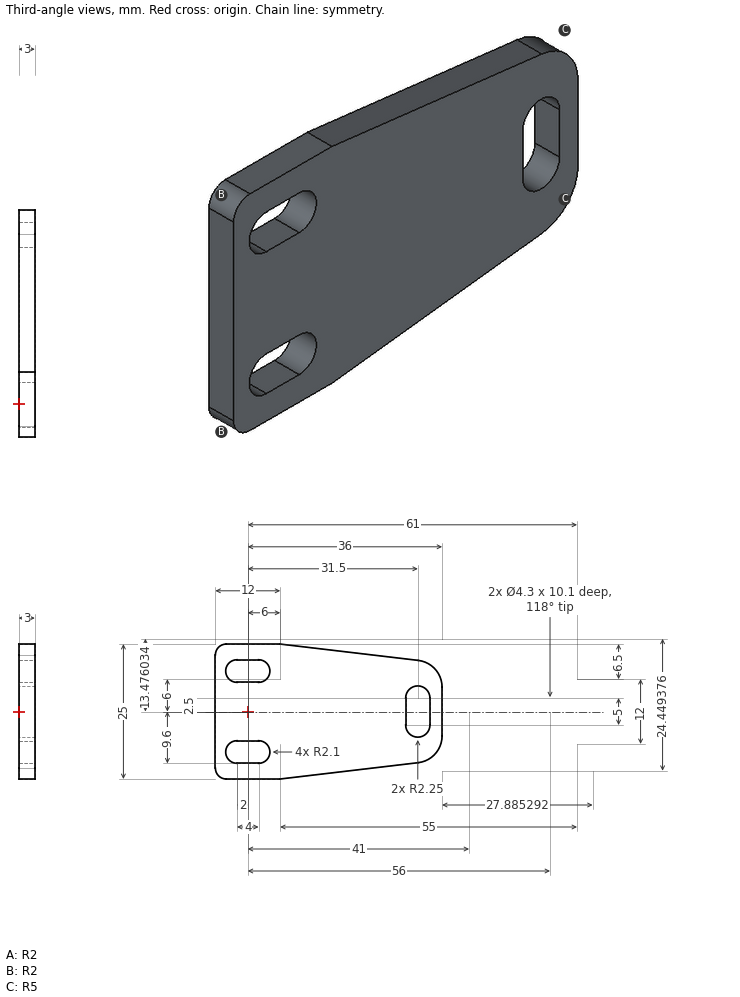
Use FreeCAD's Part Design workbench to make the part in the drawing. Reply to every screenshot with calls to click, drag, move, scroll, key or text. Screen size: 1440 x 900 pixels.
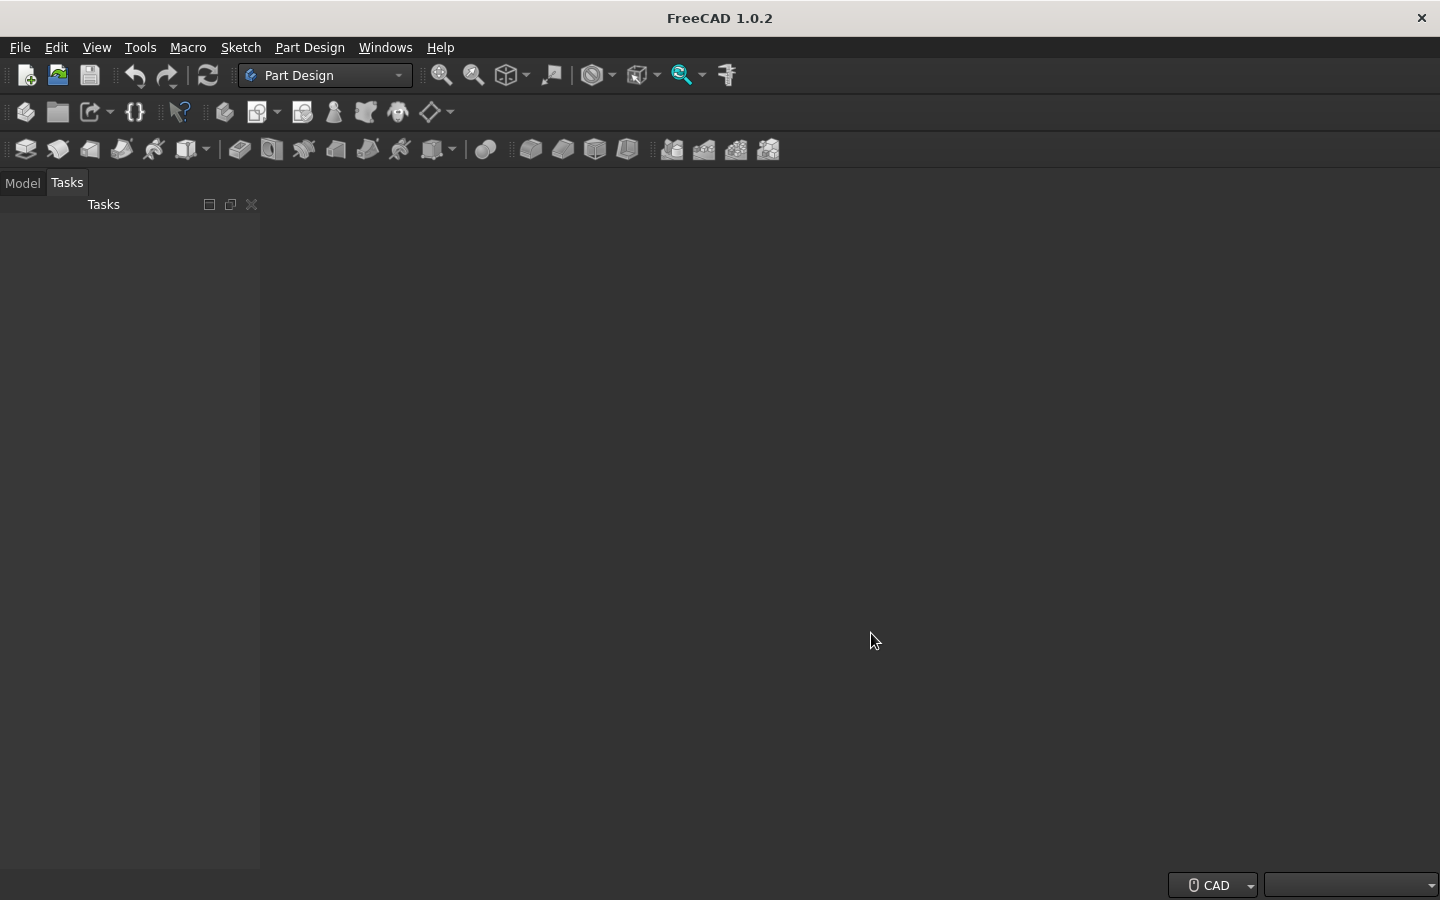
key(ctrl+n)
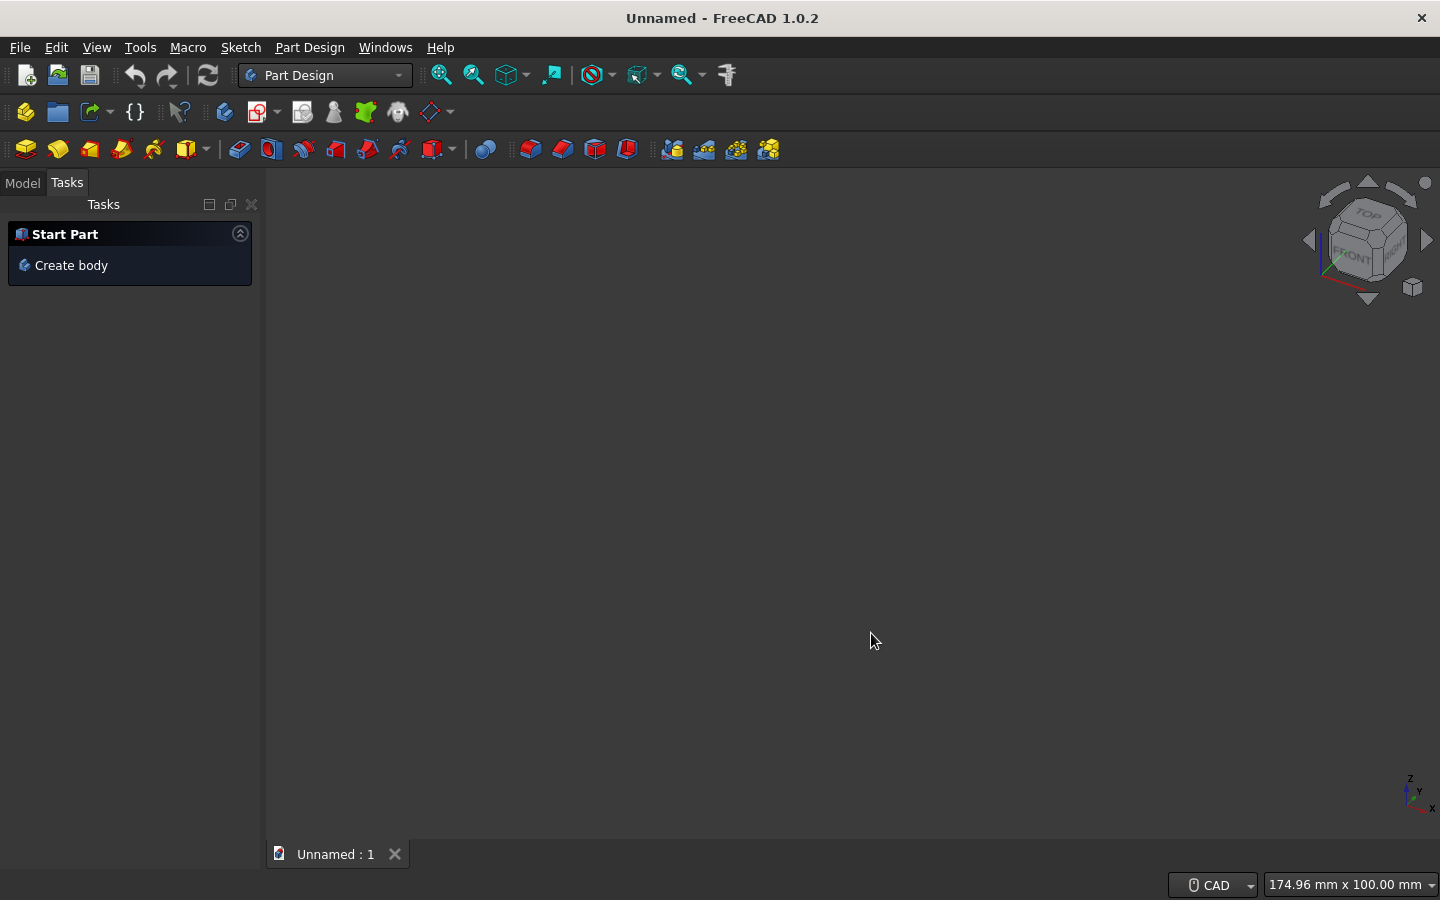
click(258, 112)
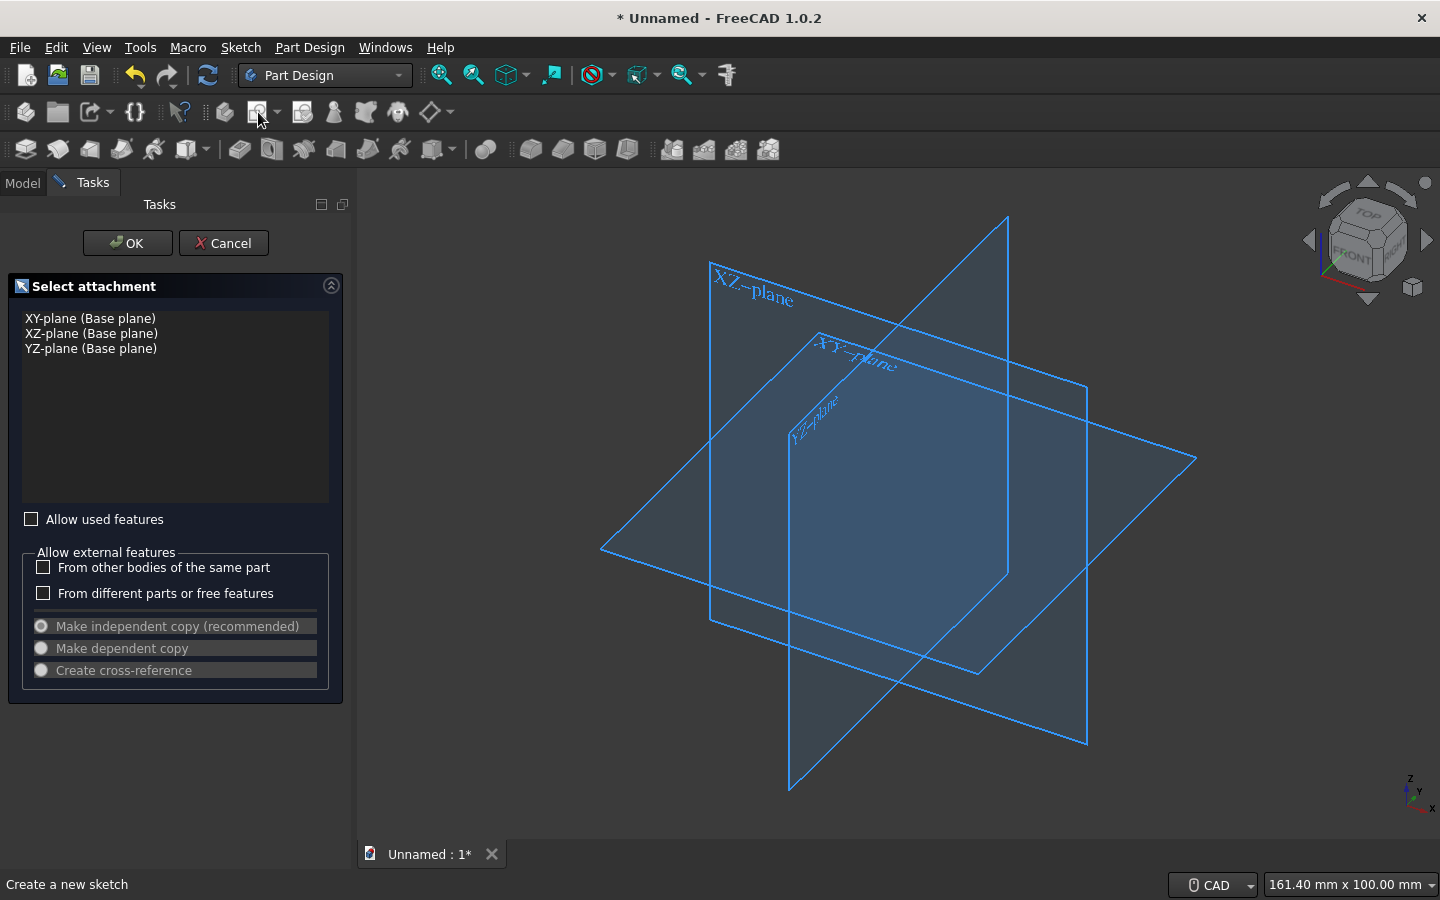
click(82, 348)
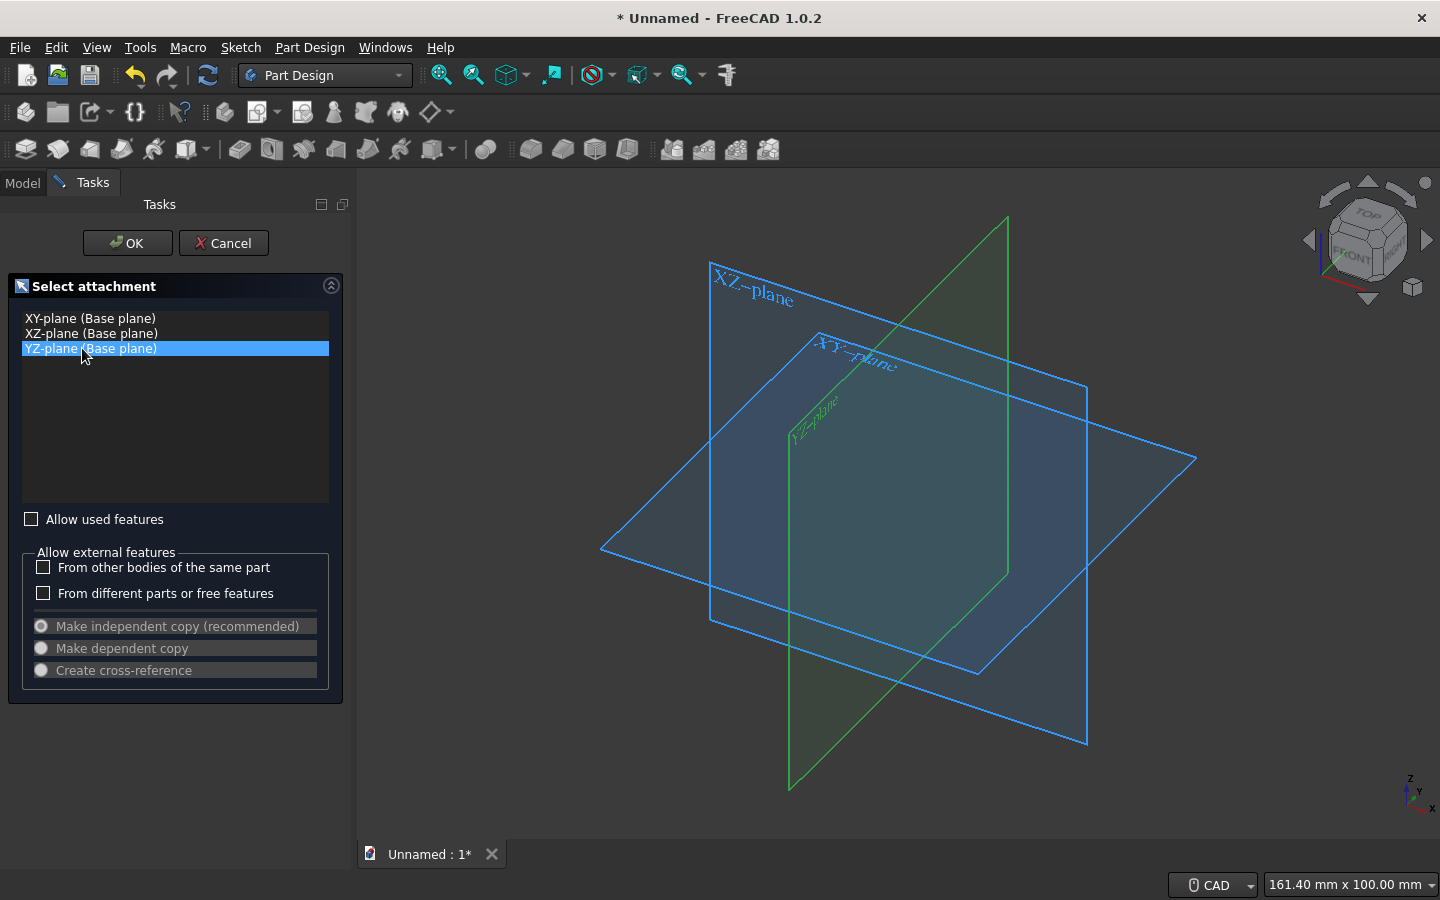
click(128, 243)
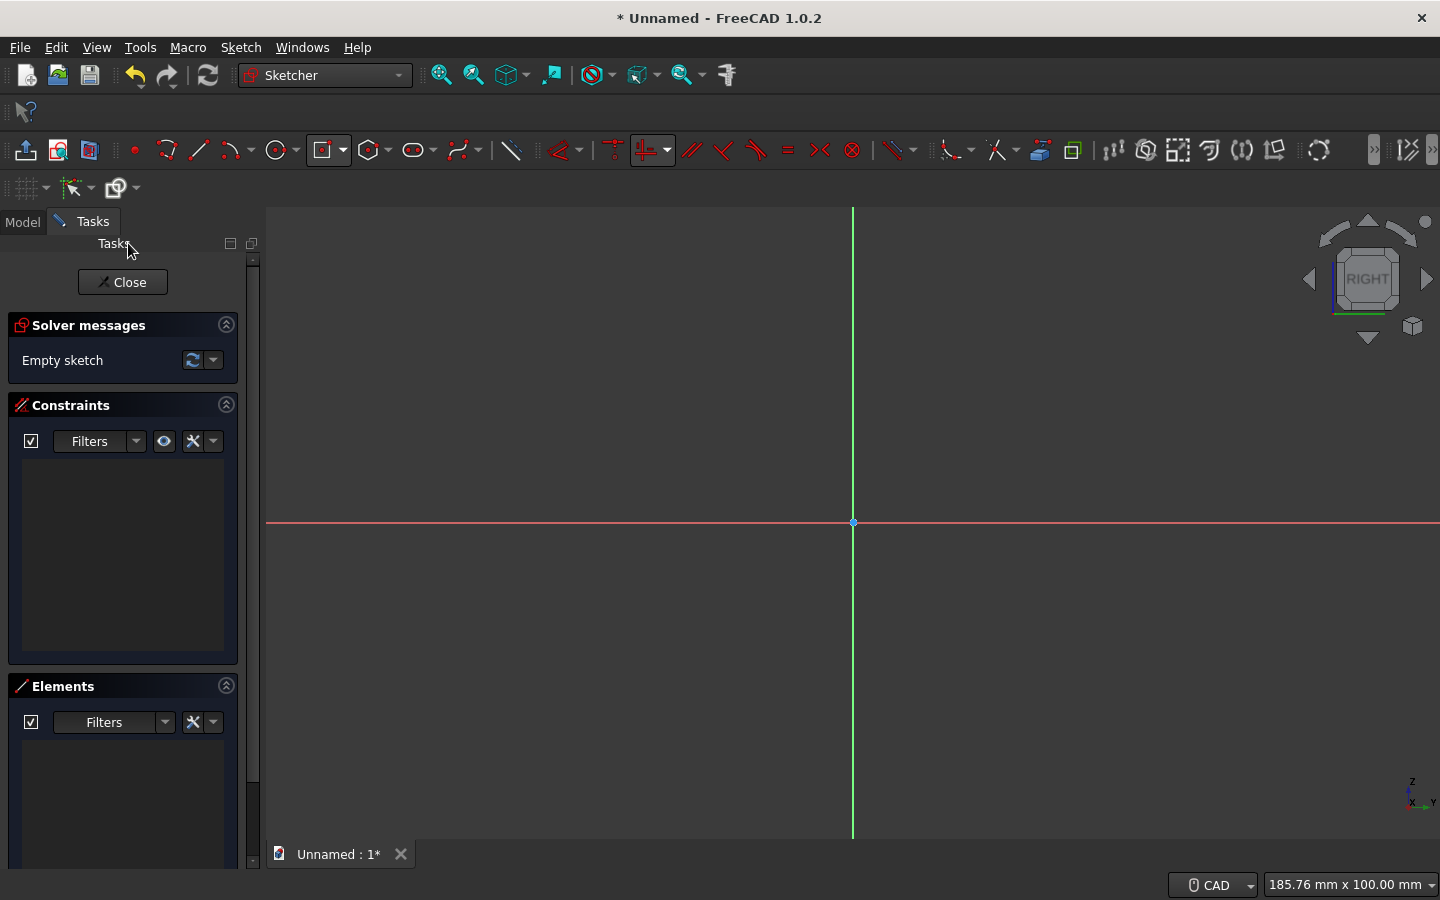
scroll(1275, 523, up, 2)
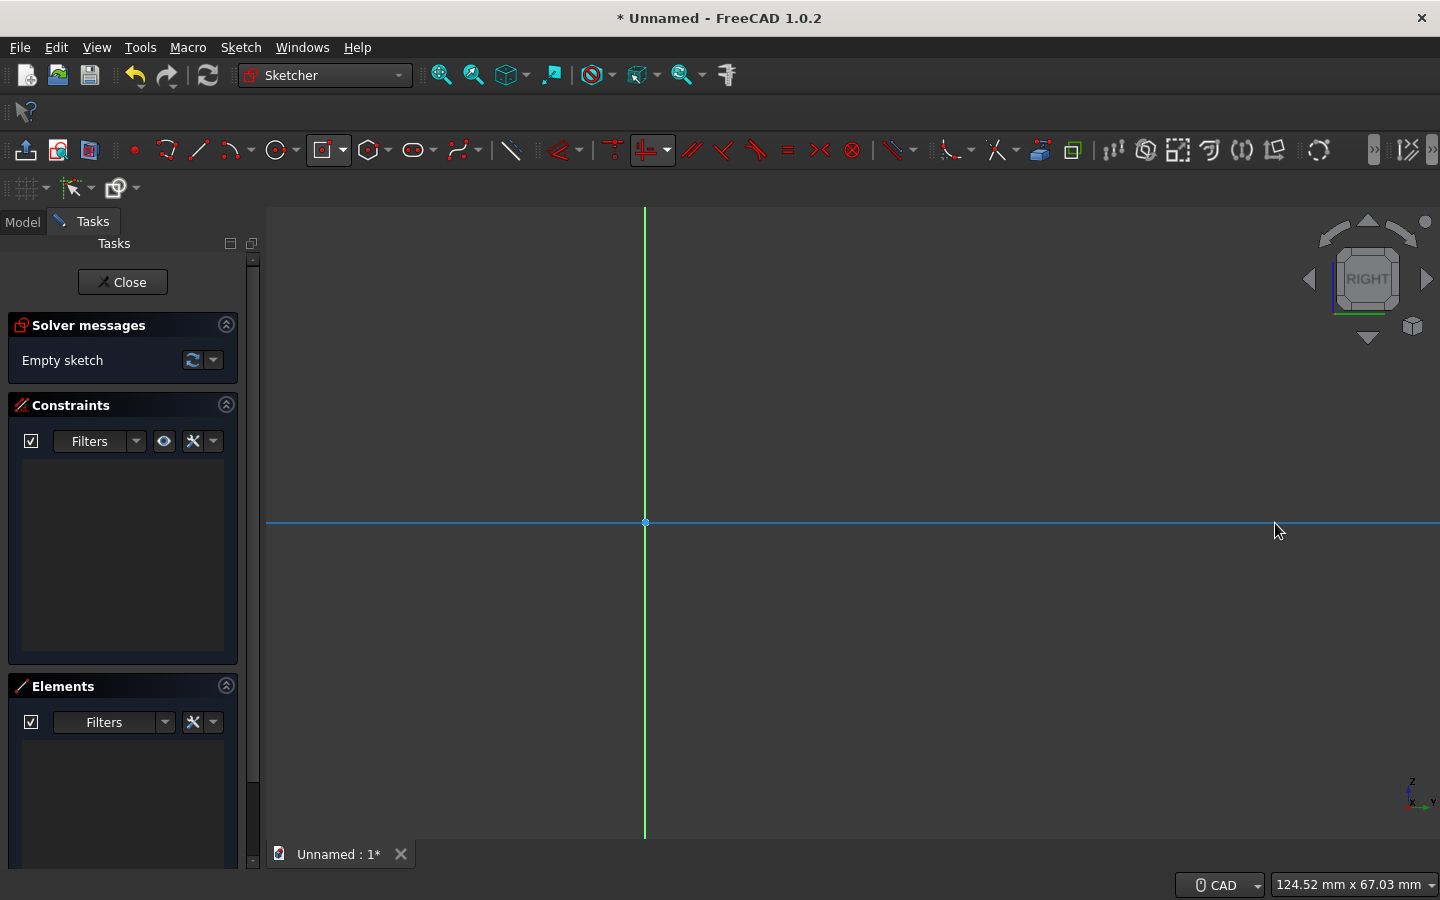
key(g)
key(m)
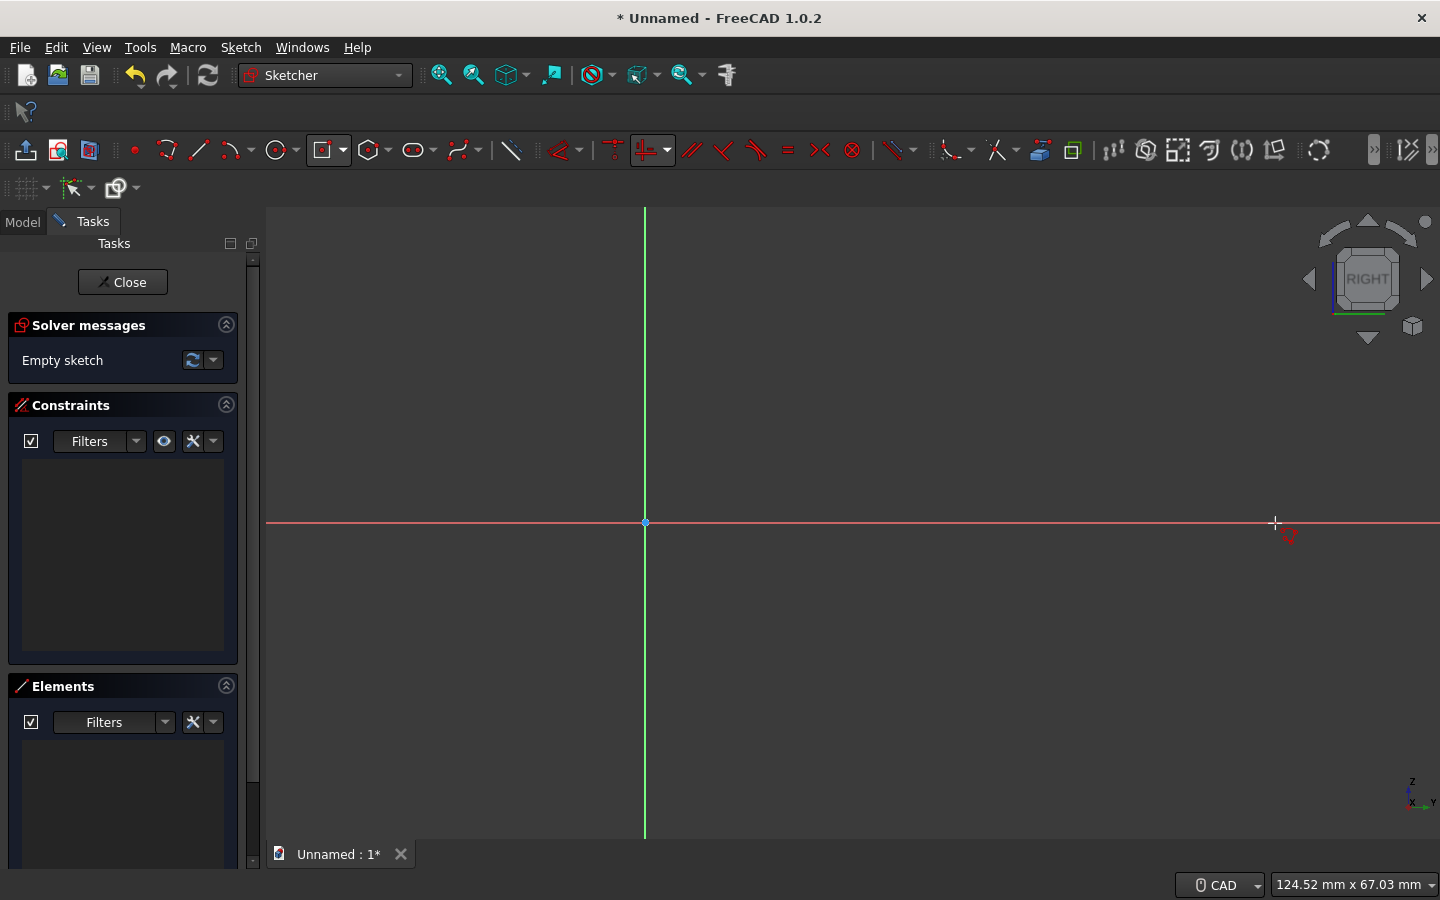
click(702, 466)
click(702, 405)
click(588, 405)
click(588, 641)
click(702, 641)
click(702, 579)
click(1220, 579)
click(1220, 466)
click(702, 467)
key(Escape)
key(Escape)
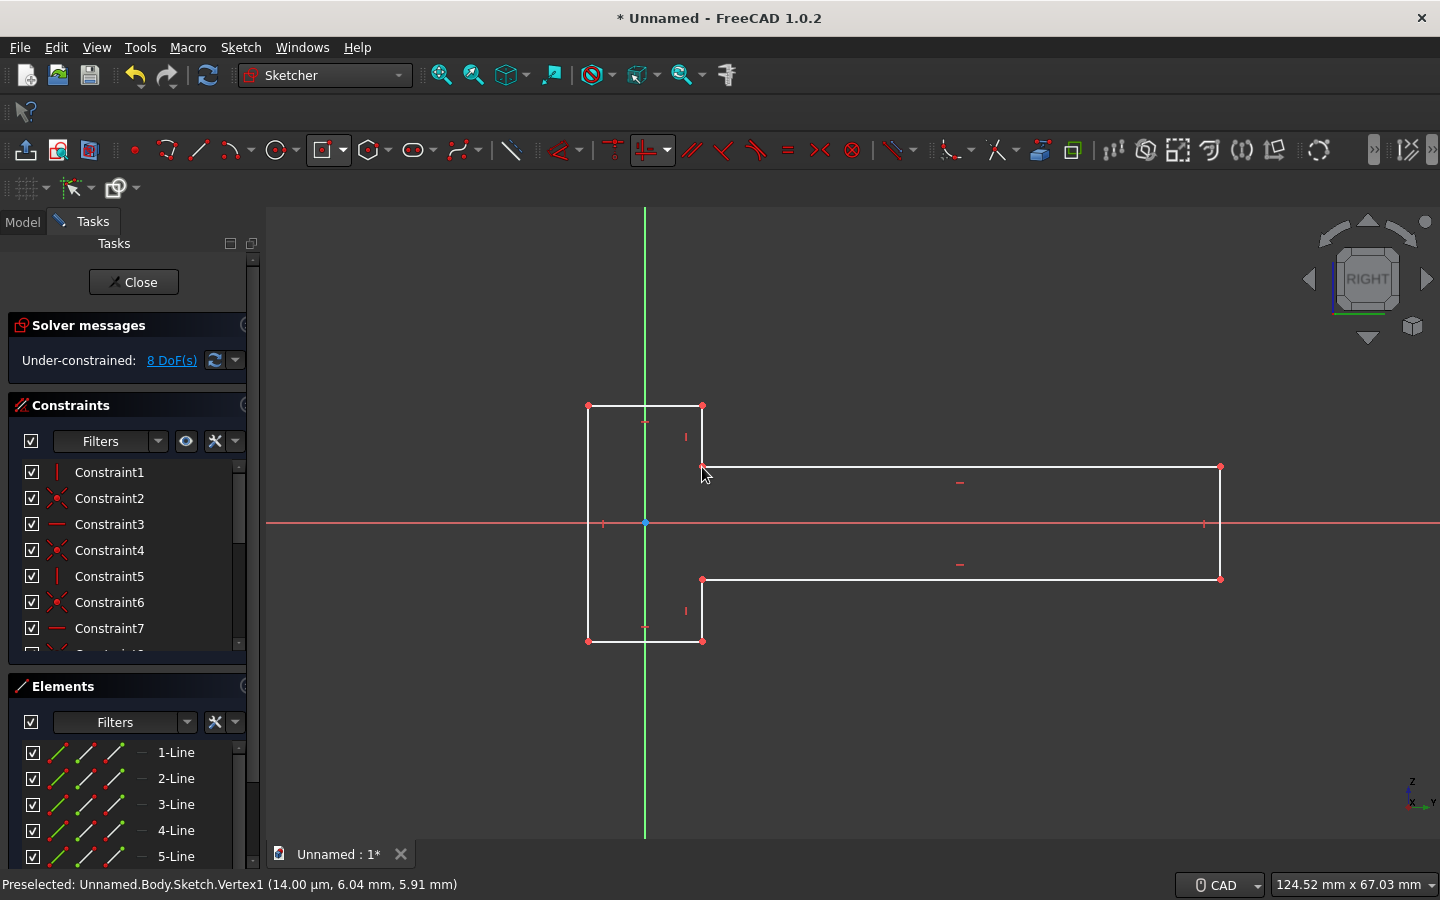
click(702, 406)